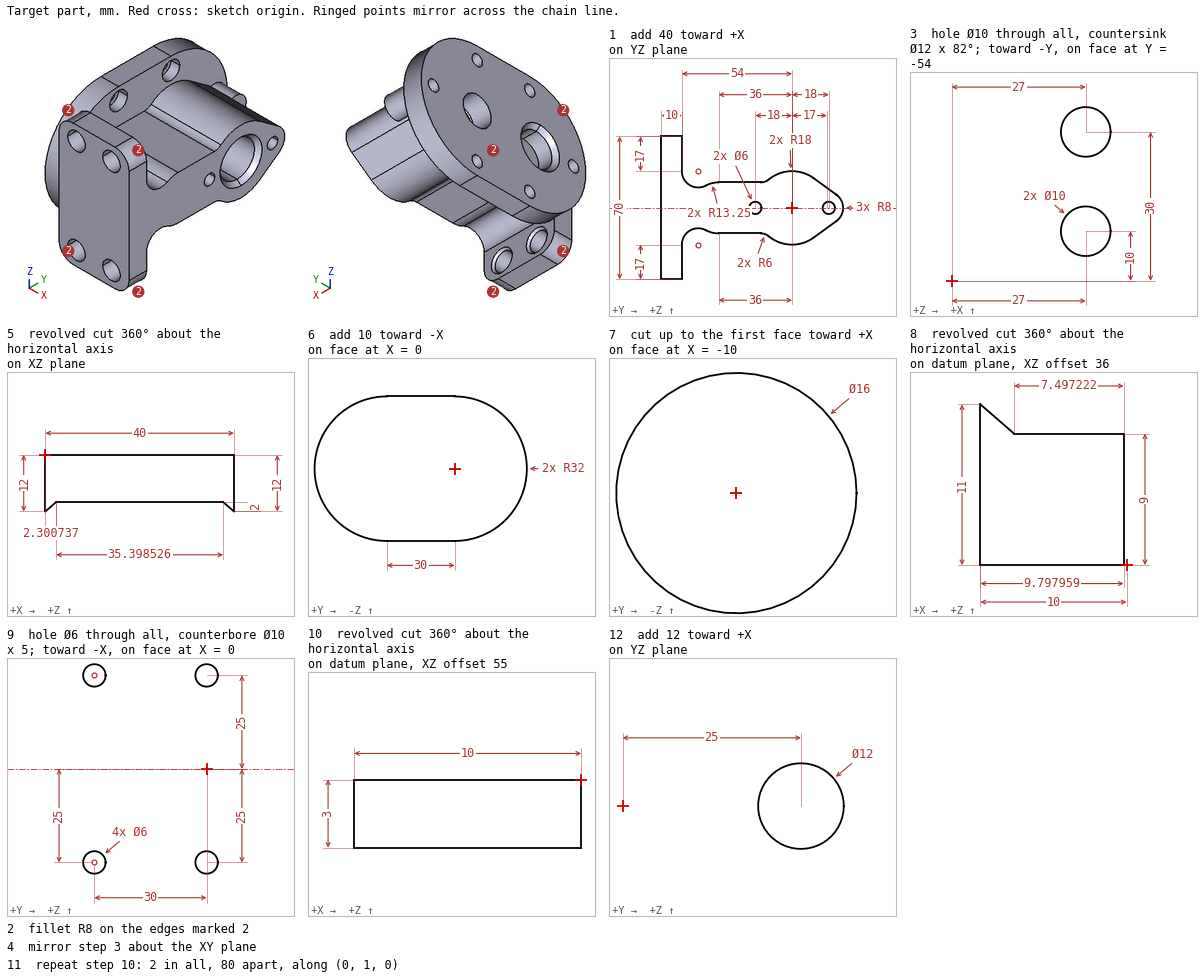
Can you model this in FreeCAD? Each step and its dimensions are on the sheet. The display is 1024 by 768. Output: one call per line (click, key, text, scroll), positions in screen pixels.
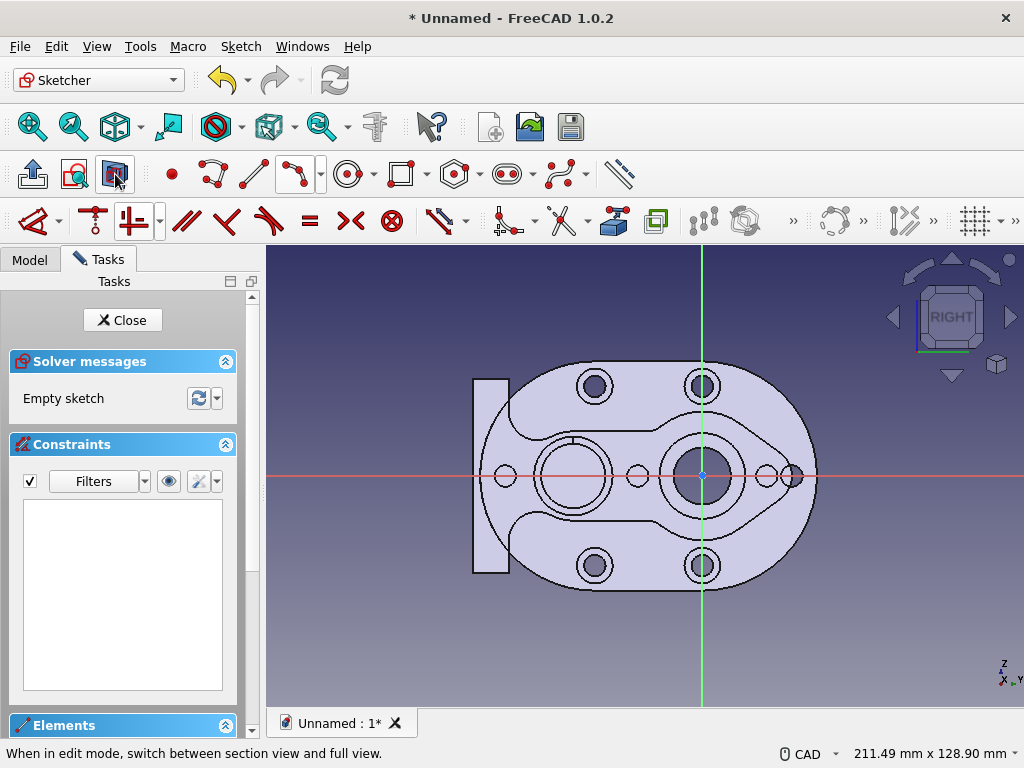
scroll(835, 476, up, 9)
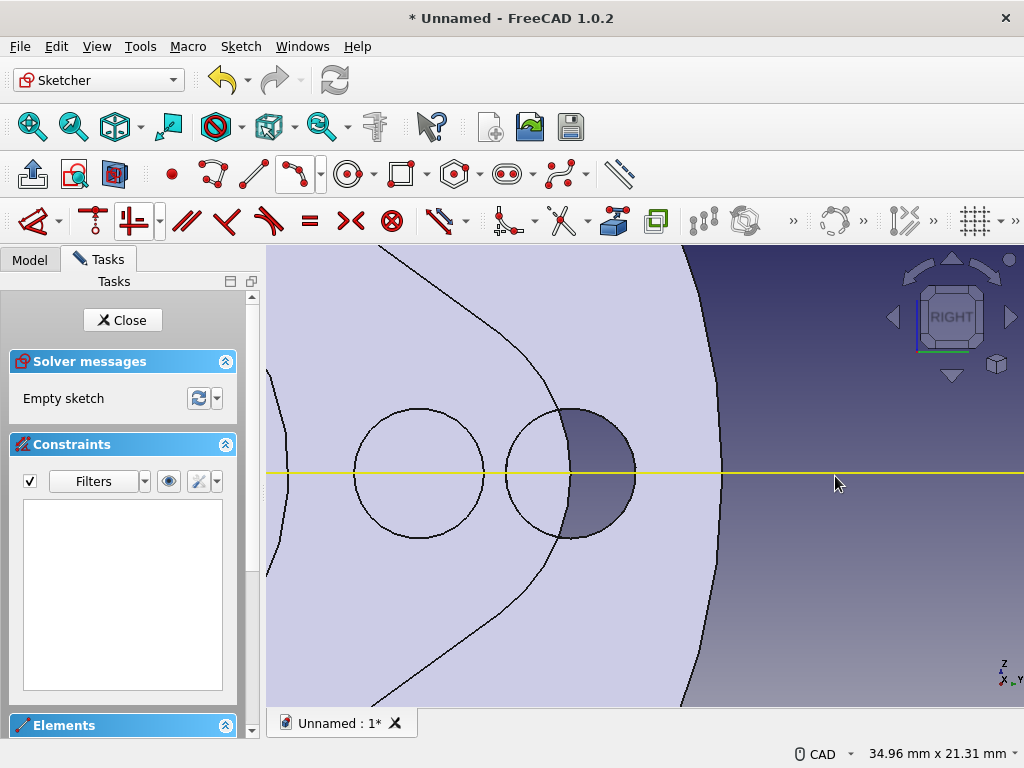
click(348, 174)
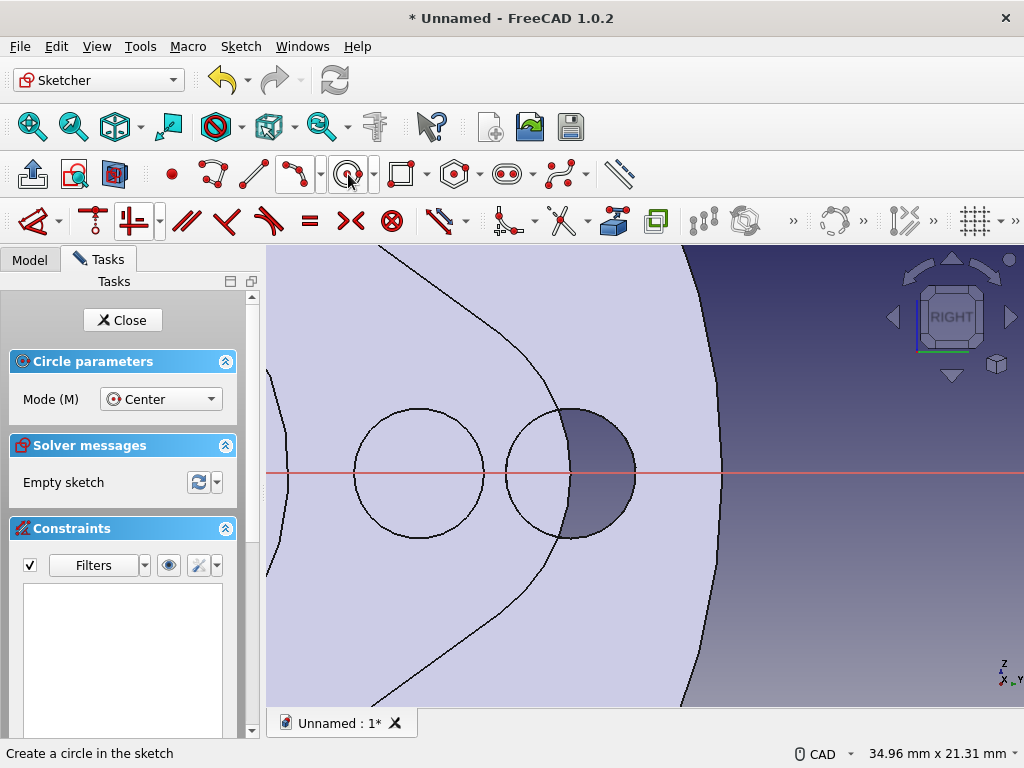
click(571, 473)
click(663, 381)
key(Escape)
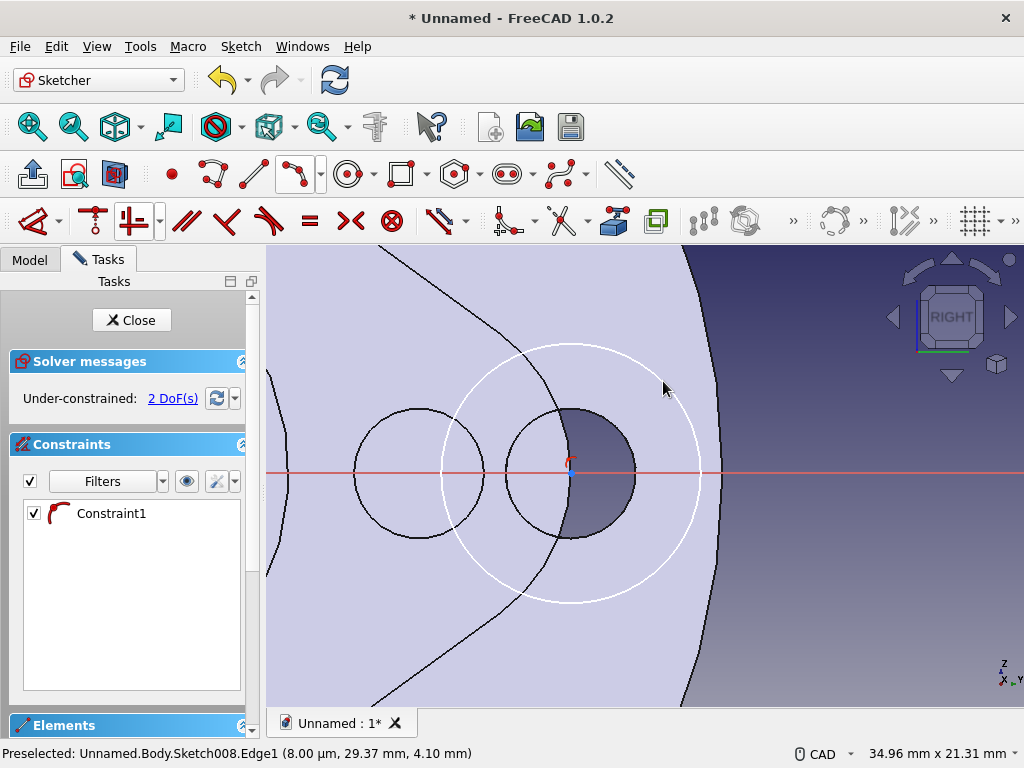
click(32, 222)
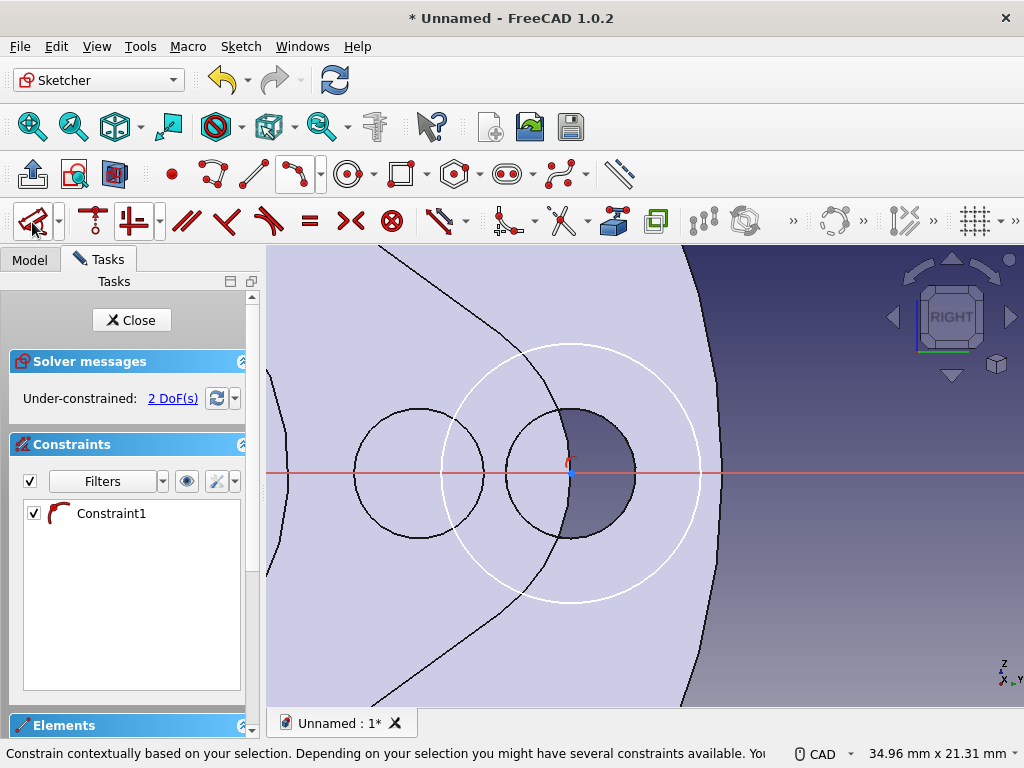
click(662, 381)
click(684, 358)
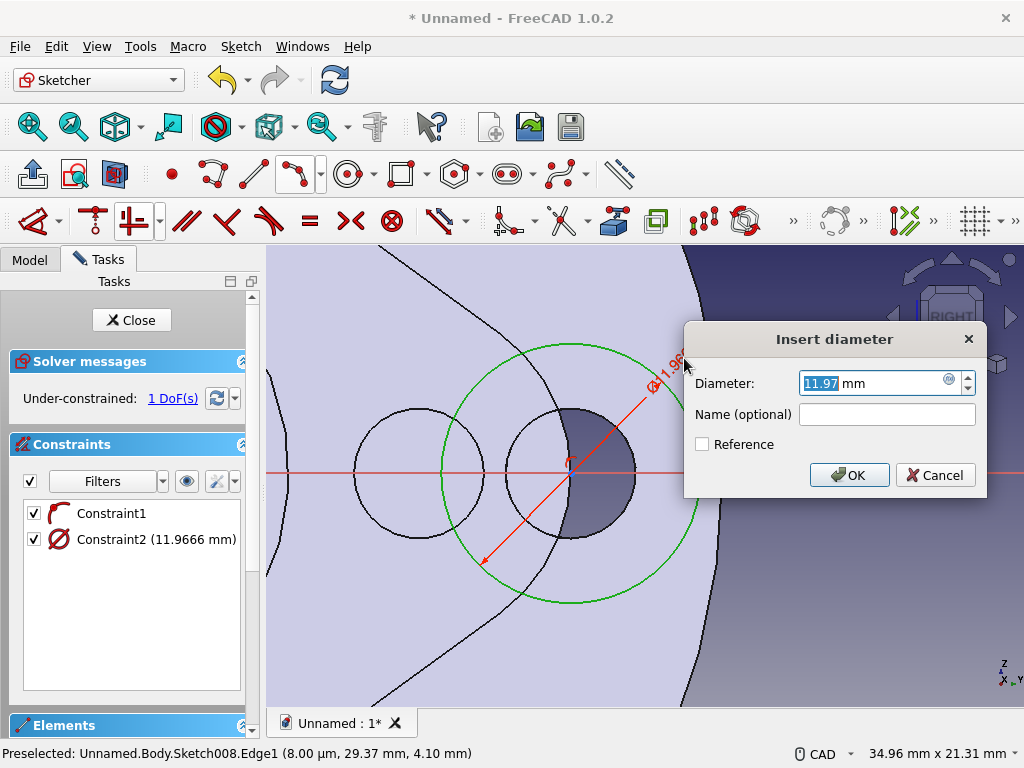
text(12)
key(Return)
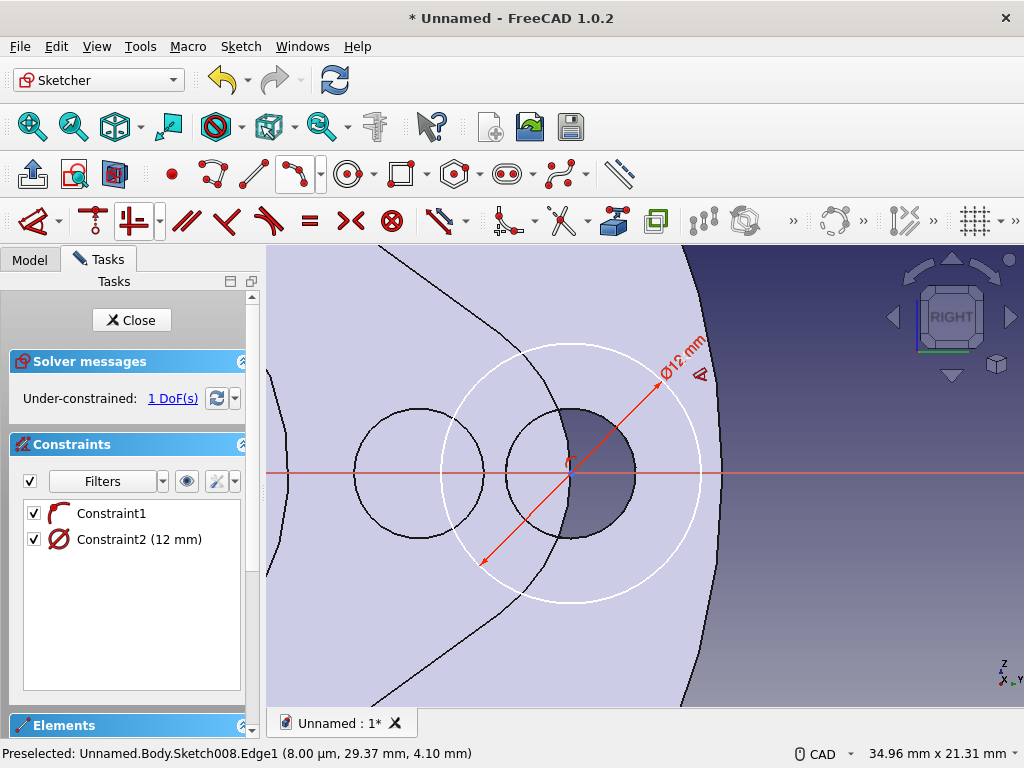
click(571, 473)
click(369, 507)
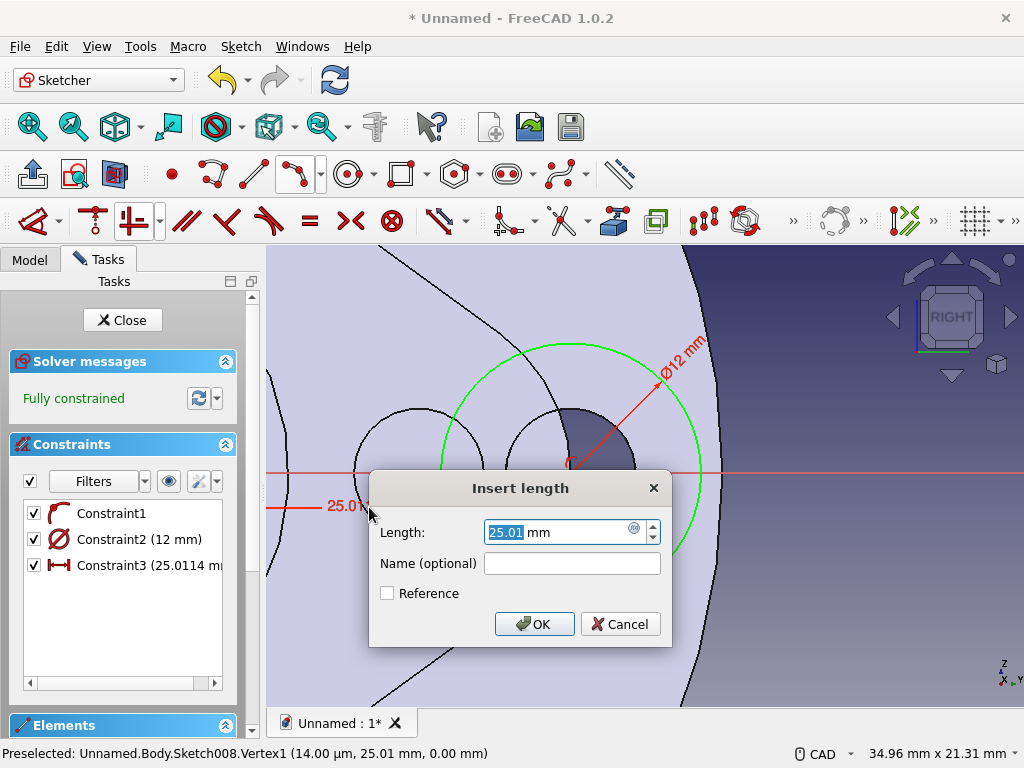
text(25)
key(Return)
key(Escape)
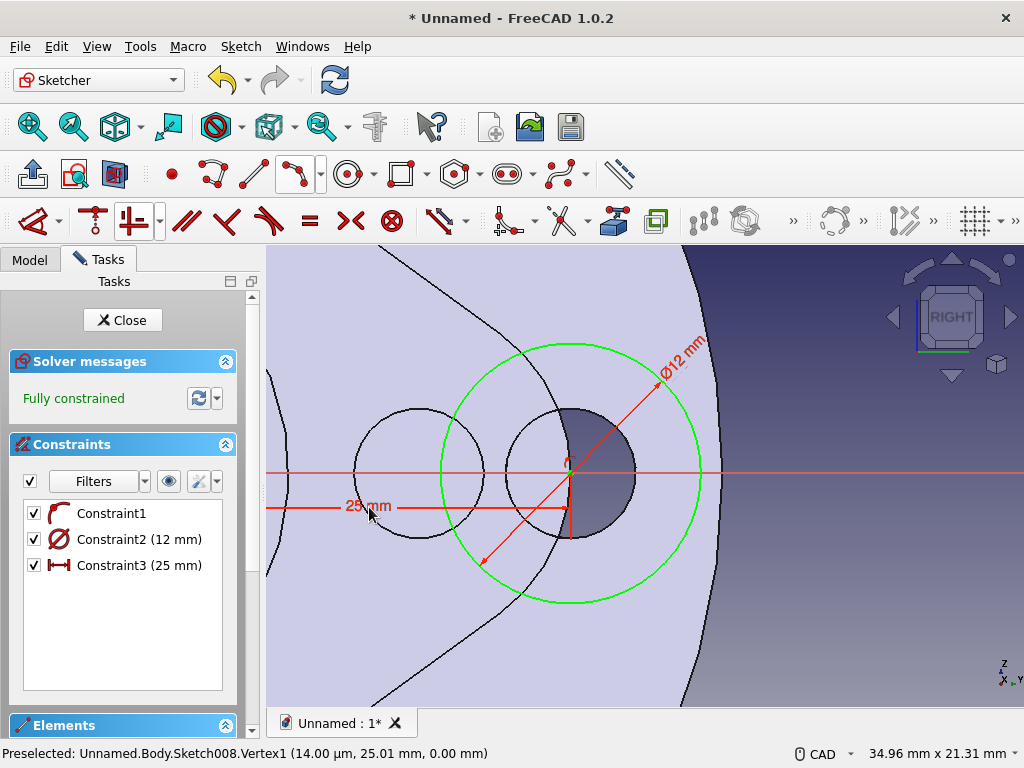
click(123, 320)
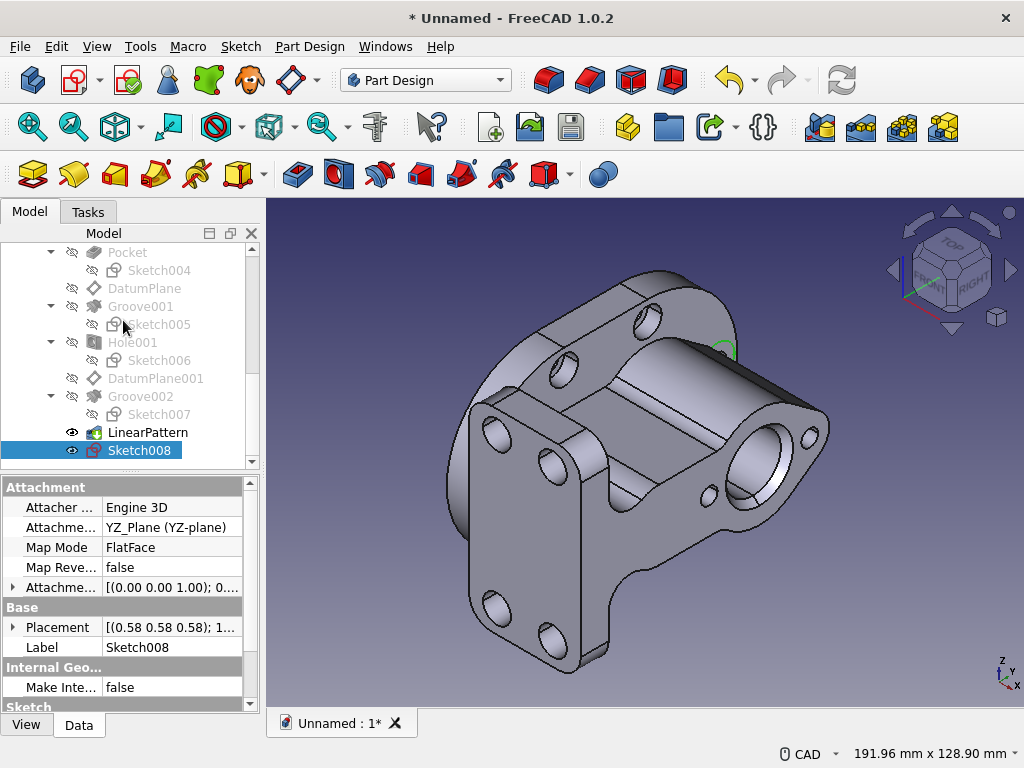
click(33, 174)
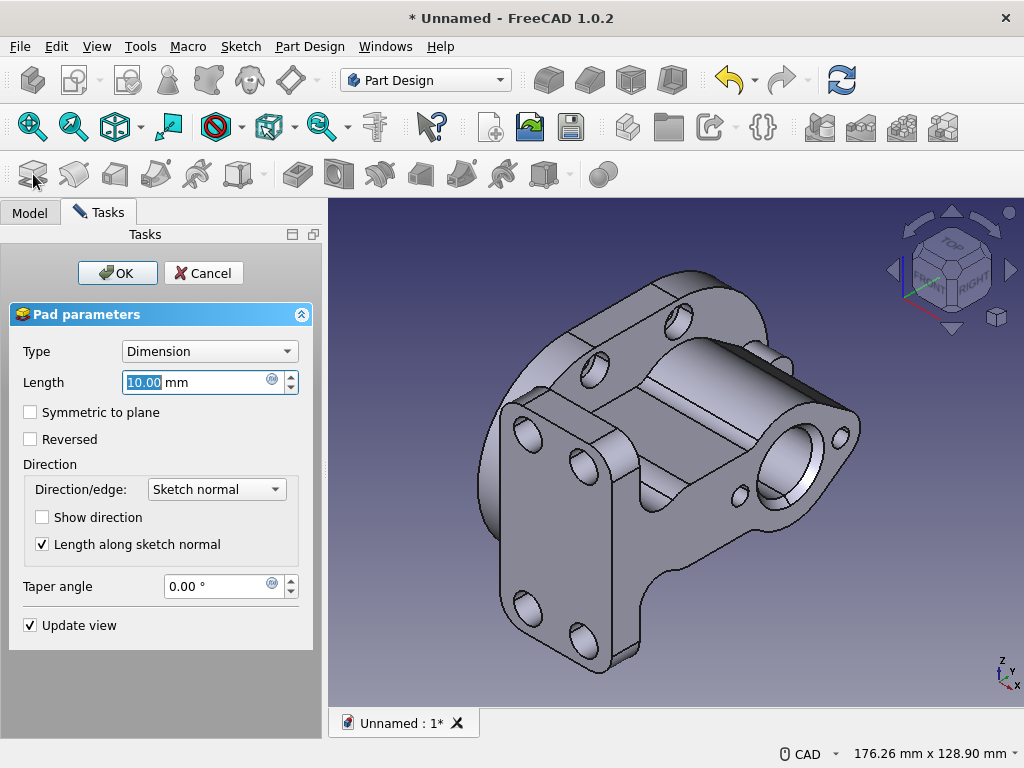
text(12)
key(Tab)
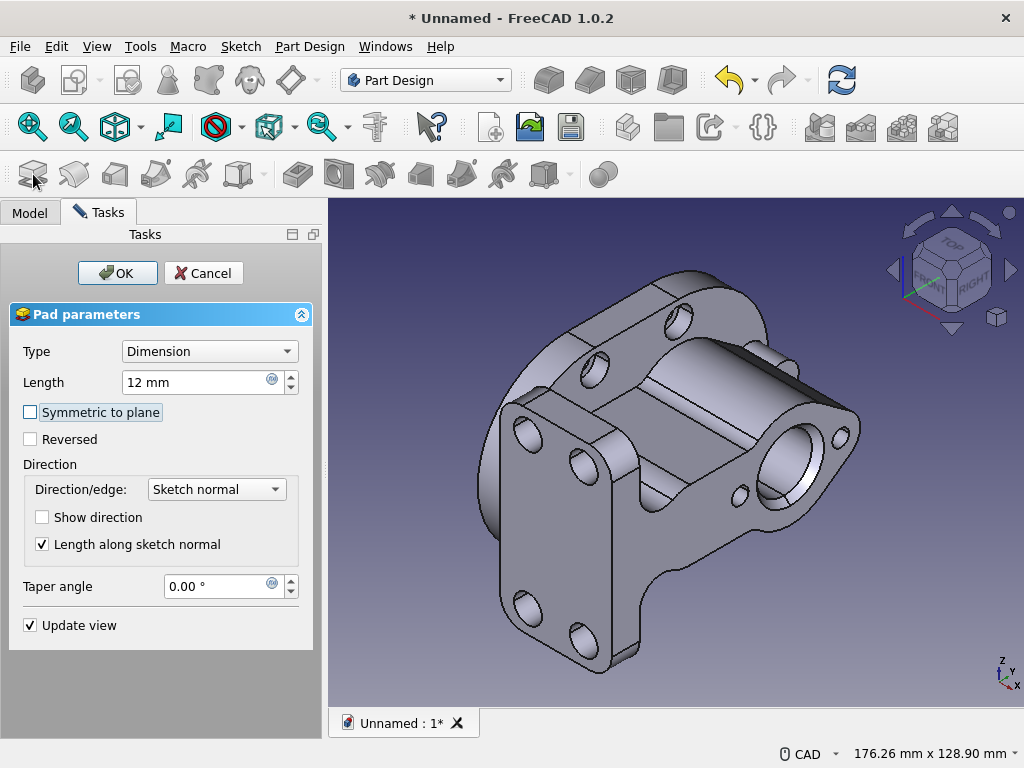
click(118, 273)